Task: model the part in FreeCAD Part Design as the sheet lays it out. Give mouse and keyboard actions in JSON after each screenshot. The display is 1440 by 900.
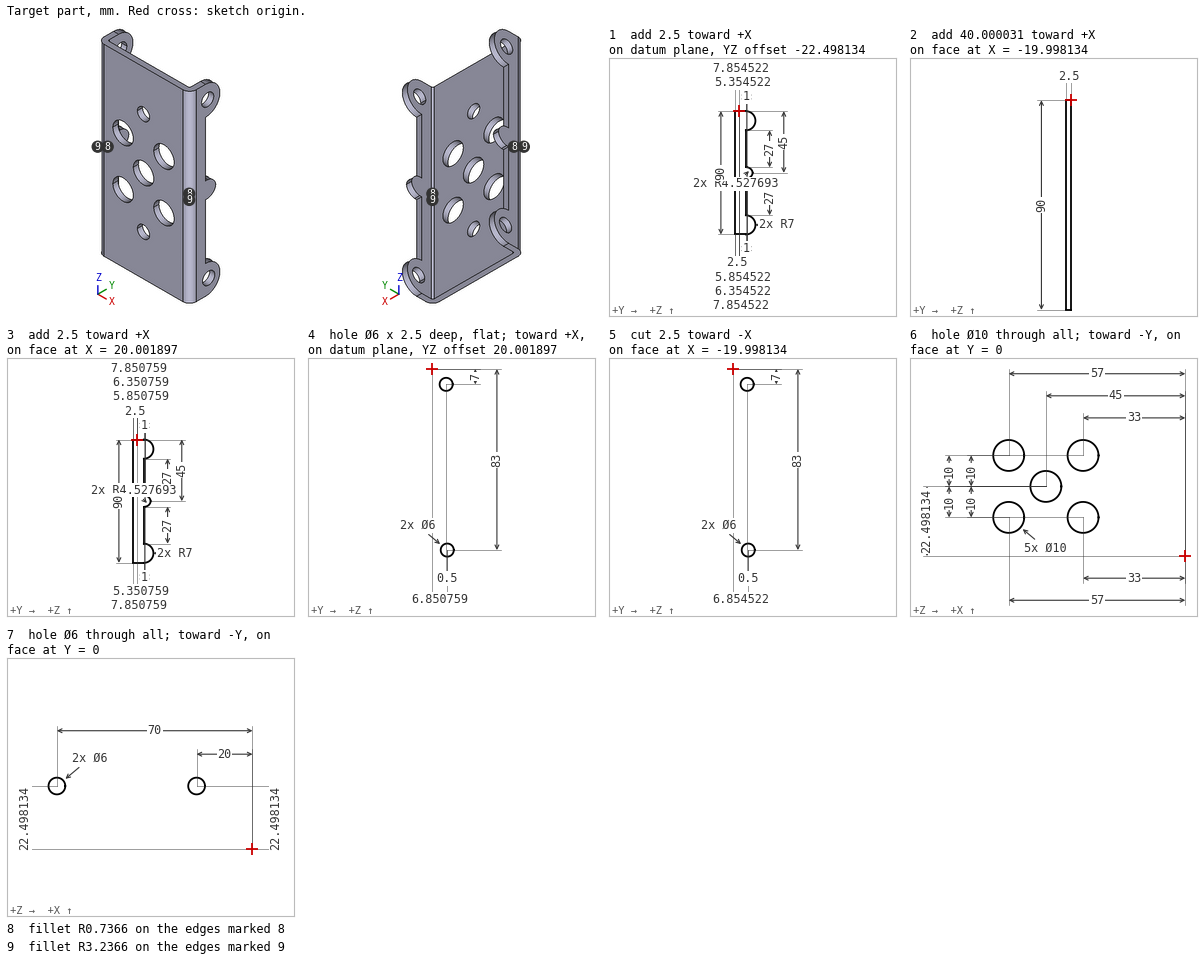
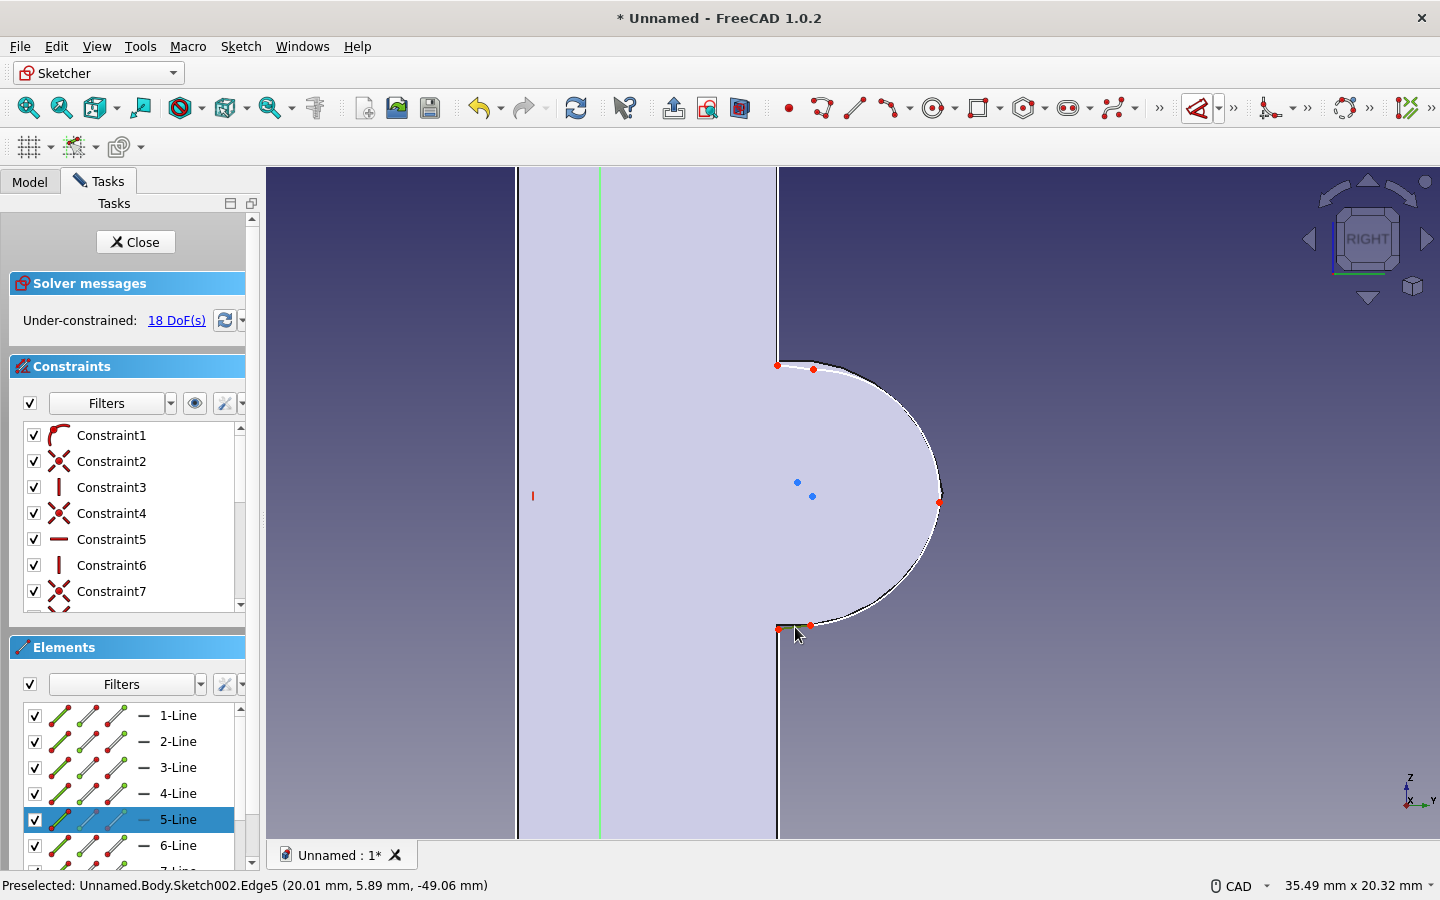
{"action": "key", "text": "h"}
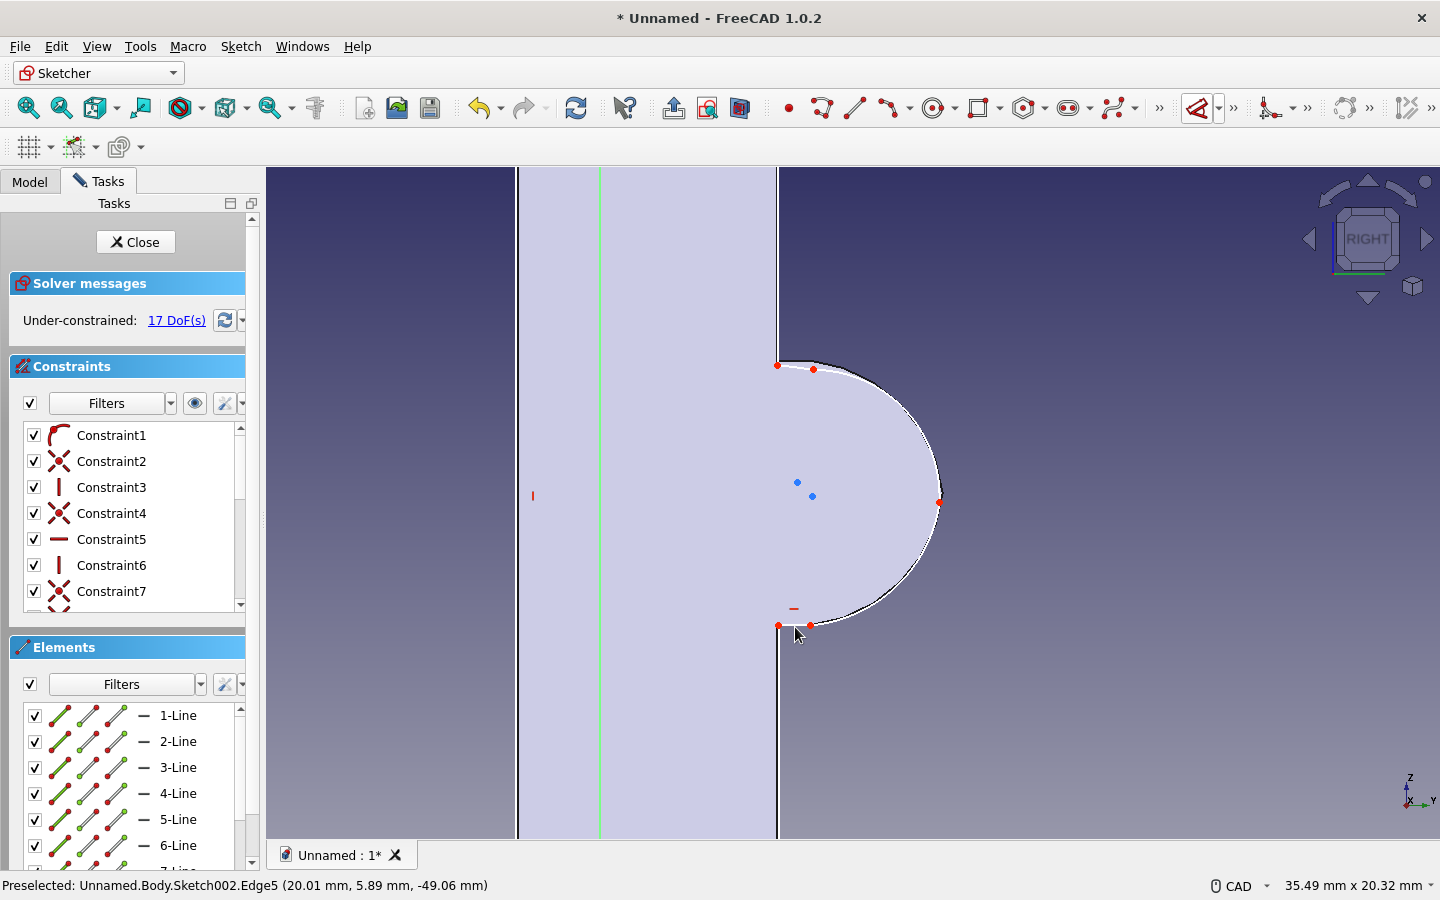
{"action": "scroll", "coordinate": [803, 368], "scroll_direction": "up", "scroll_amount": 2}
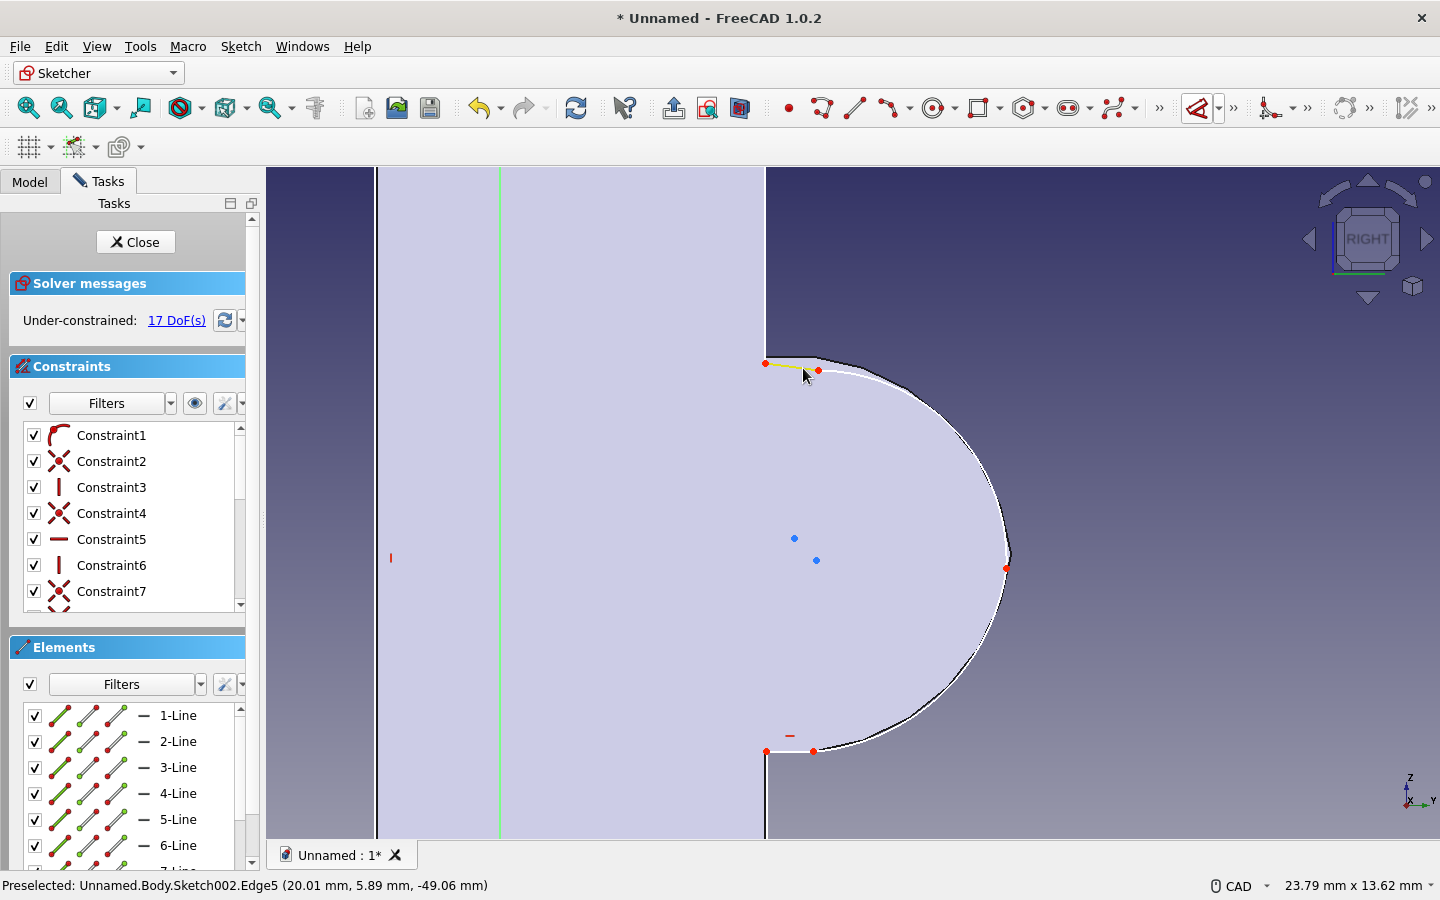
{"action": "left_click", "coordinate": [803, 368]}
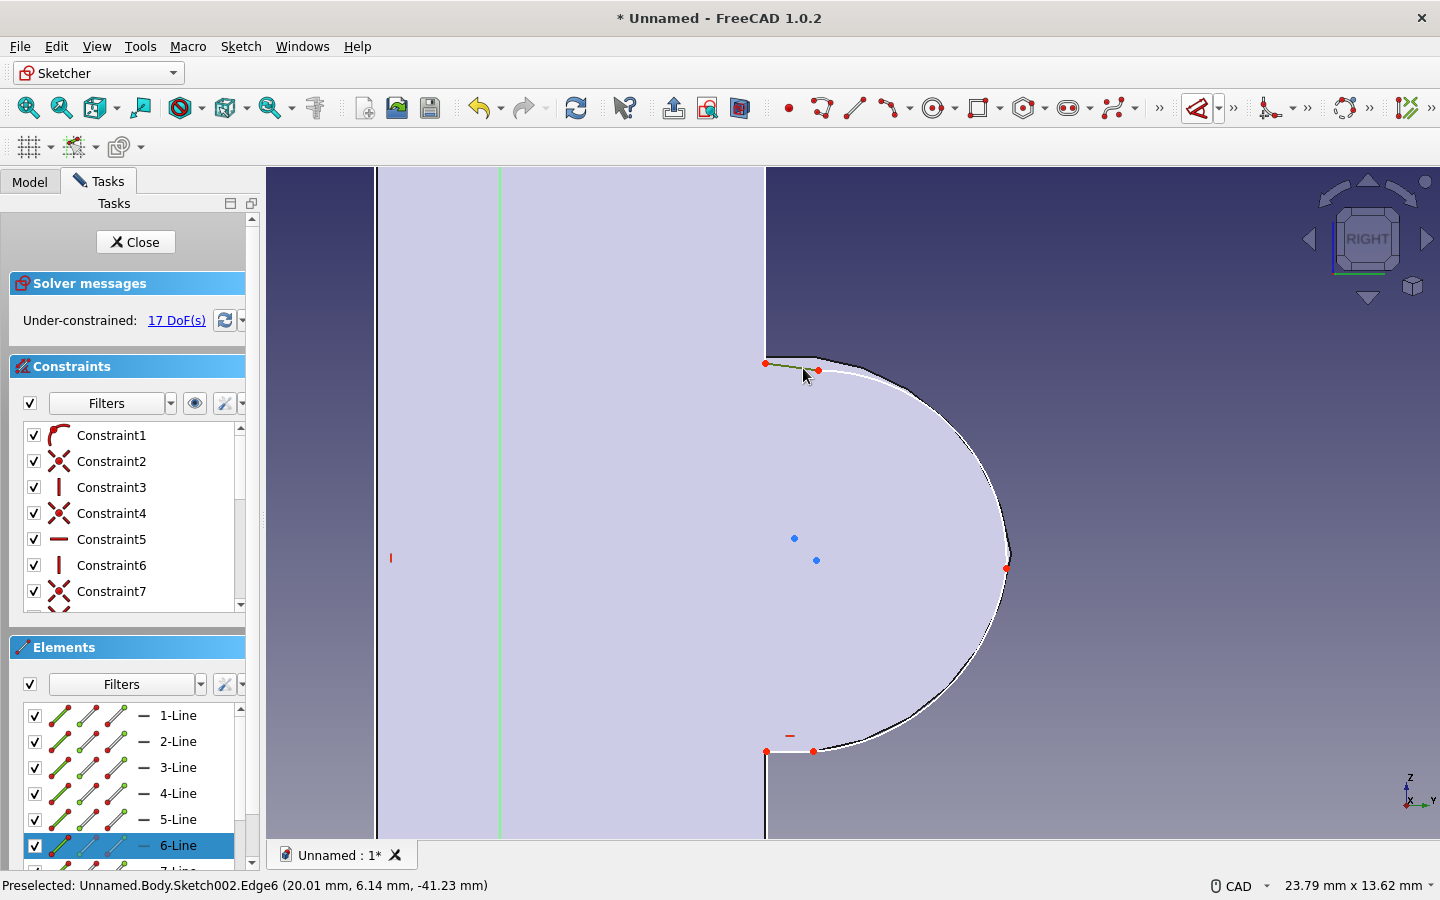
{"action": "key", "text": "h"}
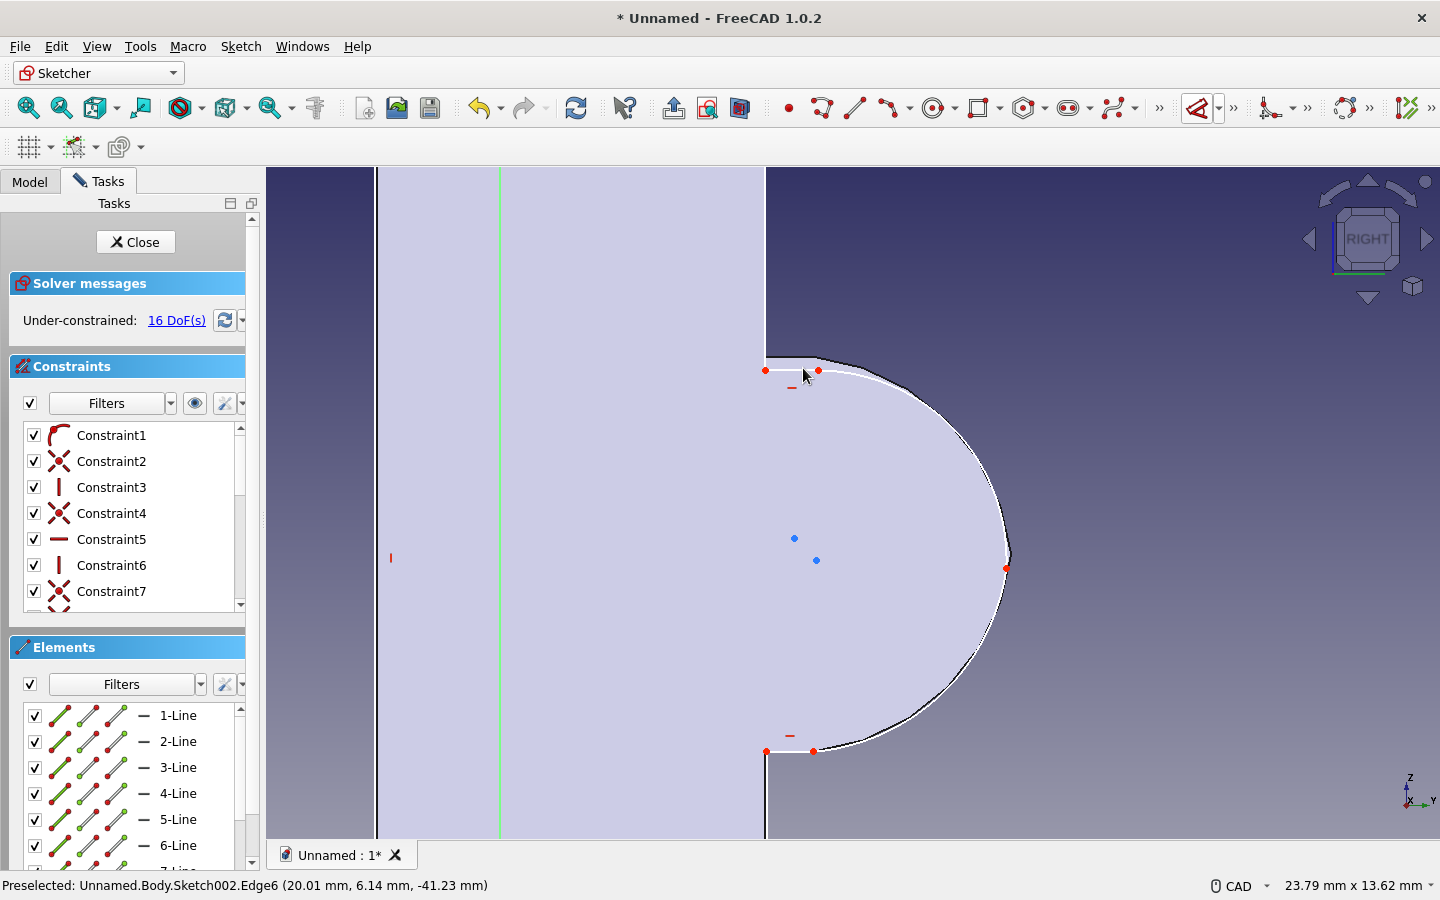
{"action": "scroll", "coordinate": [789, 498], "scroll_direction": "down", "scroll_amount": 12}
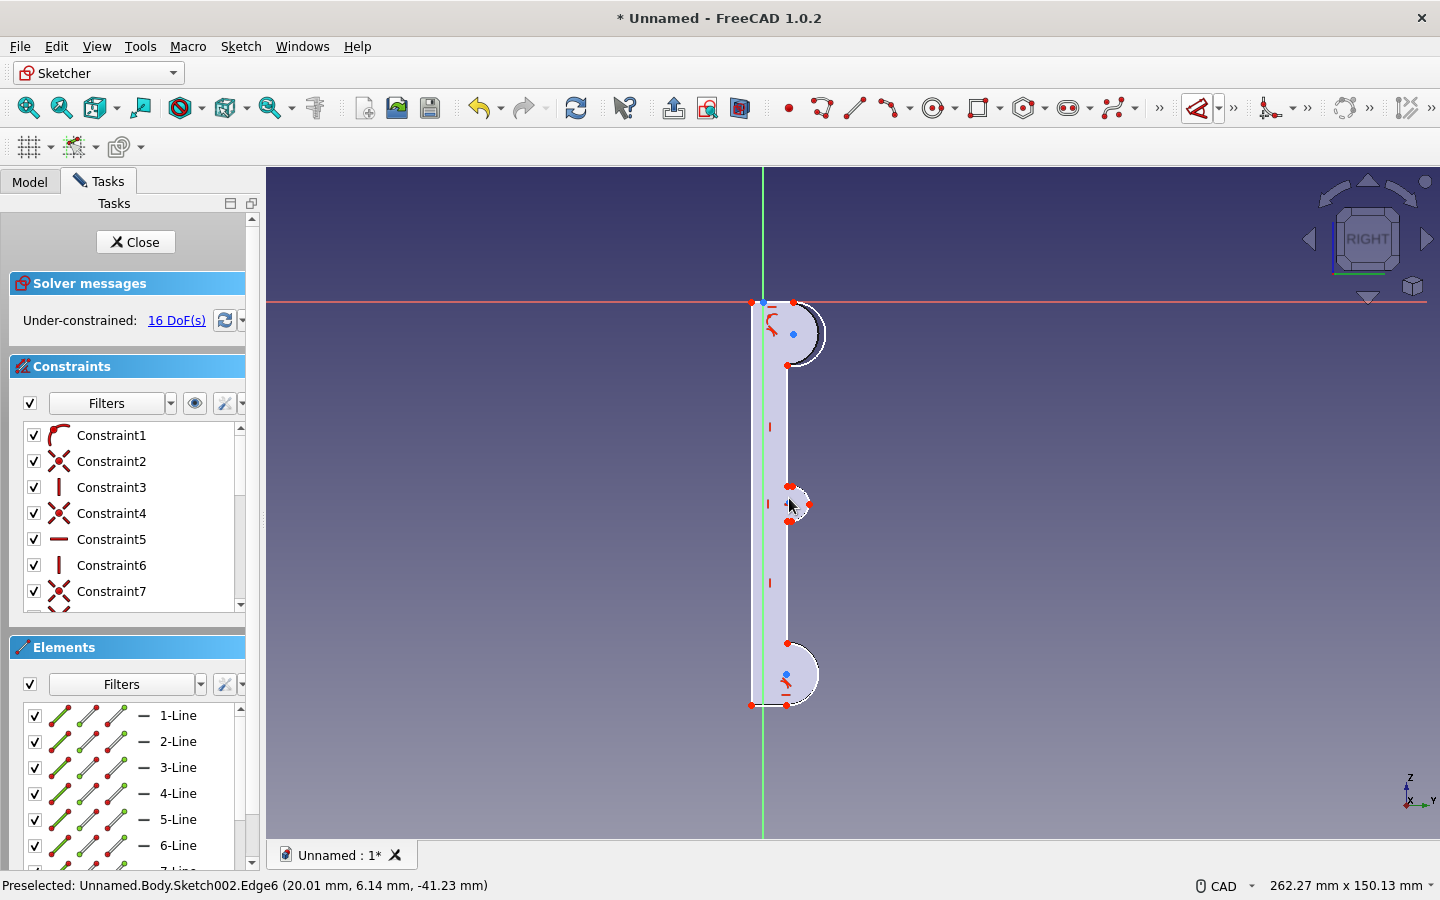
{"action": "scroll", "coordinate": [799, 519], "scroll_direction": "up", "scroll_amount": 3}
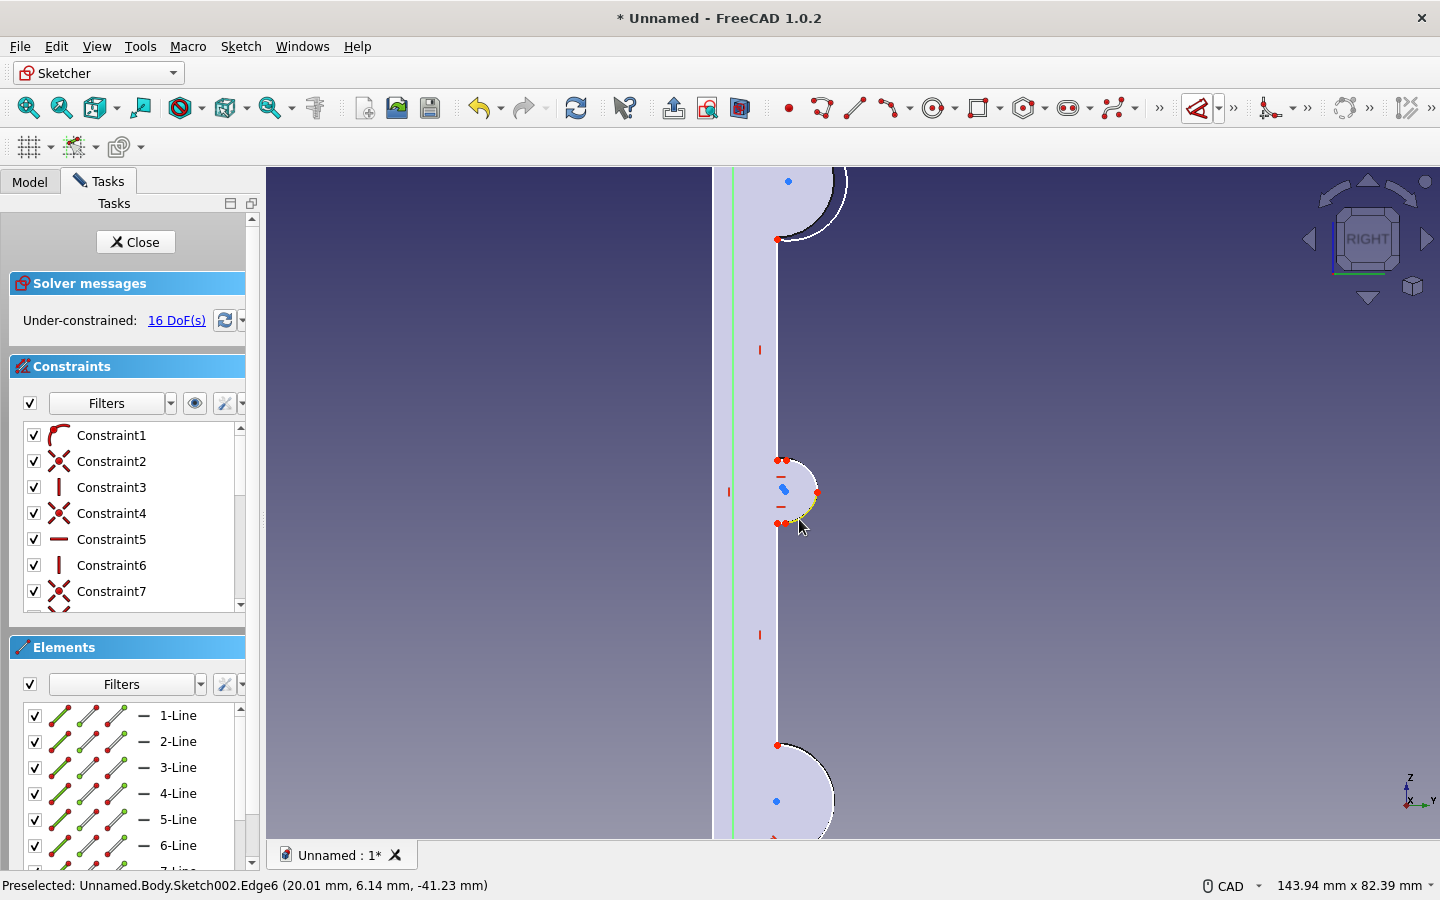
{"action": "left_click", "coordinate": [799, 519]}